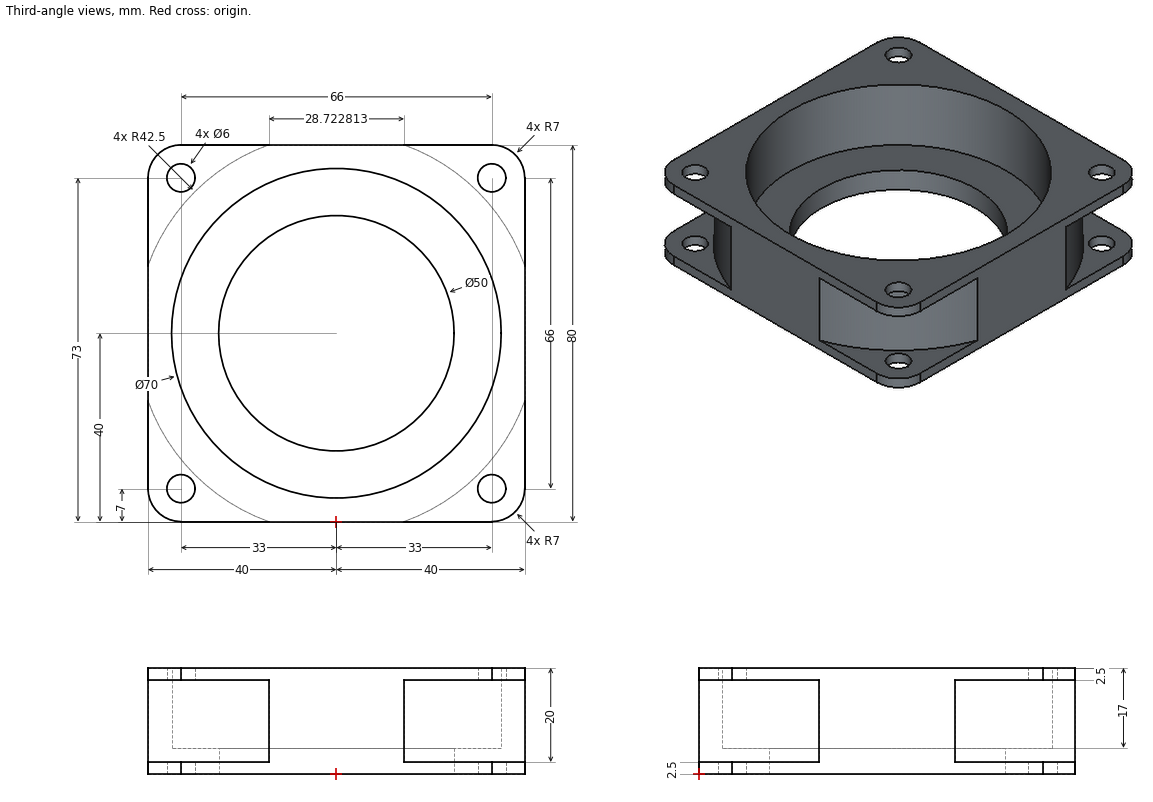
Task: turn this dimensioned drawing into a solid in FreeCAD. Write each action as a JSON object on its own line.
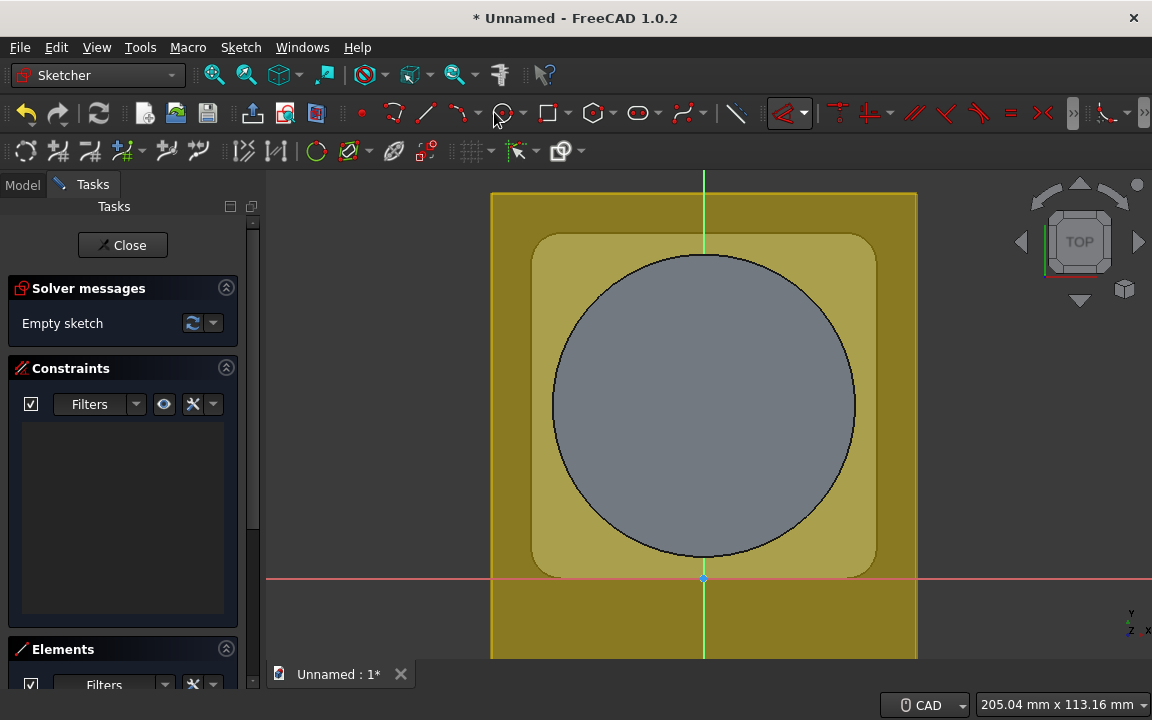
{"action": "left_click", "coordinate": [318, 114]}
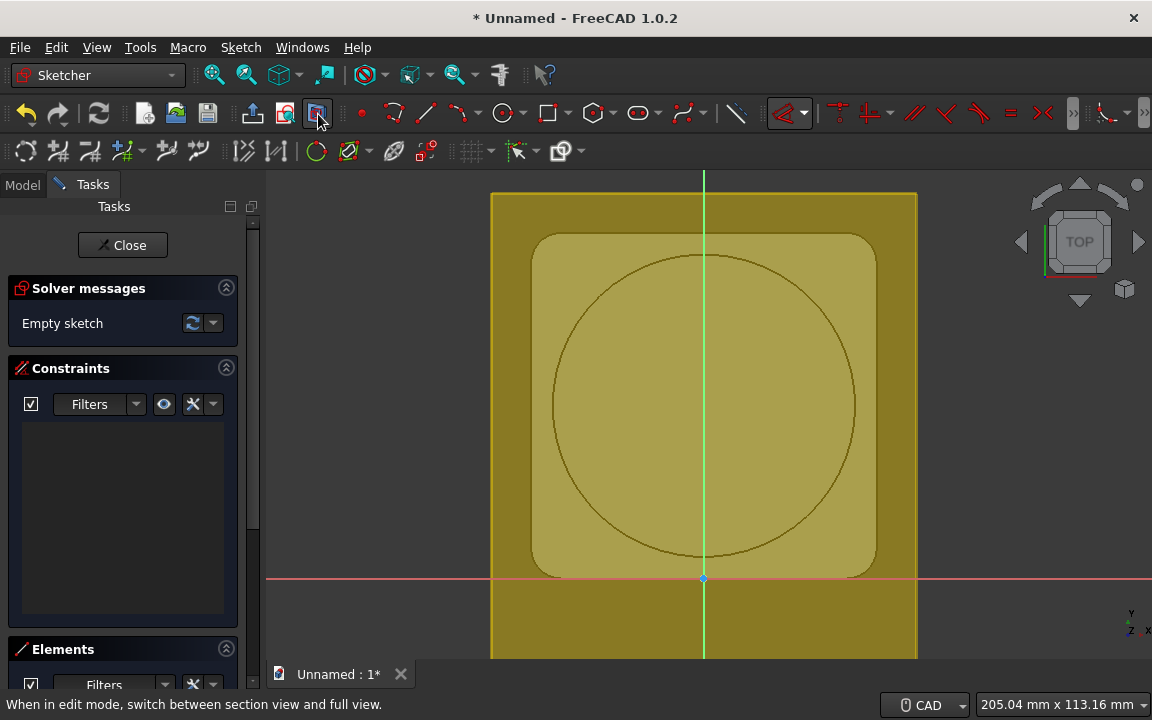
{"action": "key", "text": "g l"}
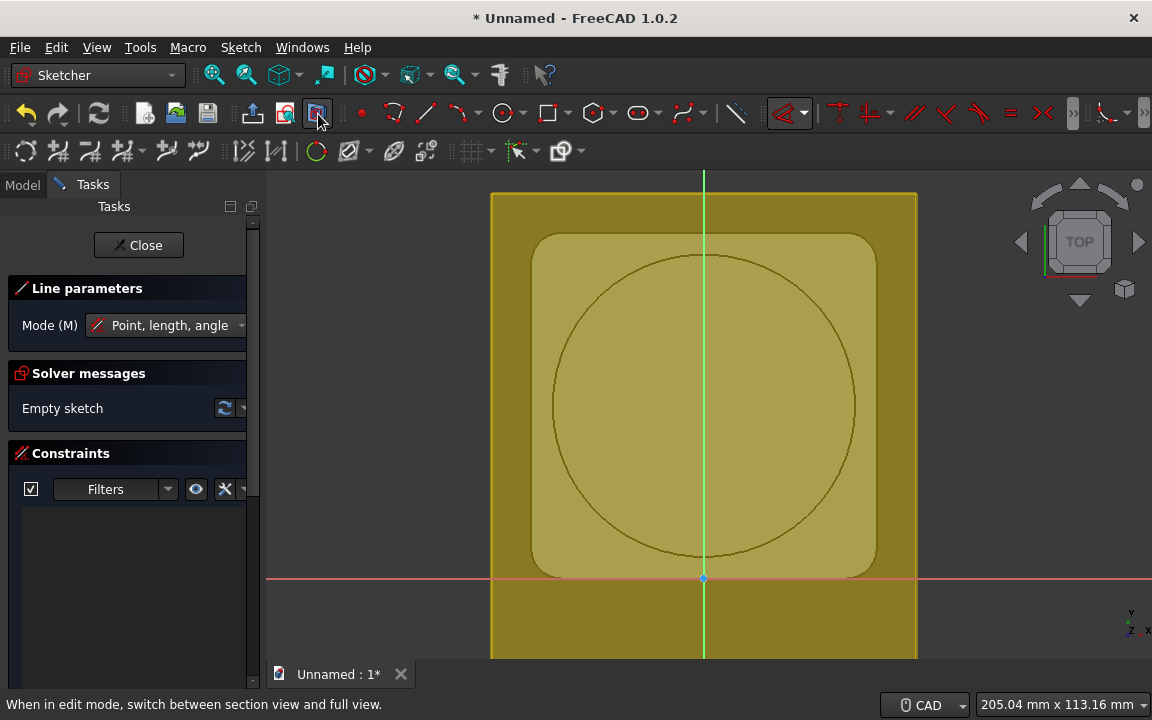
{"action": "left_click", "coordinate": [877, 548]}
{"action": "left_click", "coordinate": [877, 263]}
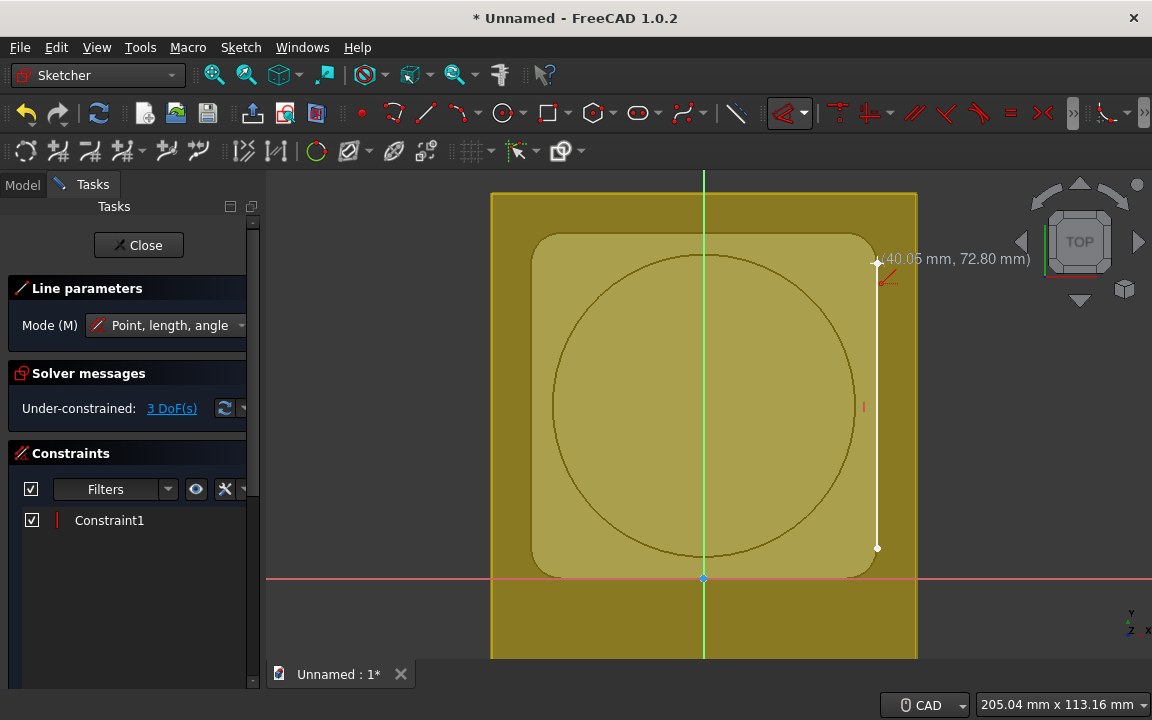
{"action": "left_click", "coordinate": [847, 233]}
{"action": "left_click", "coordinate": [561, 233]}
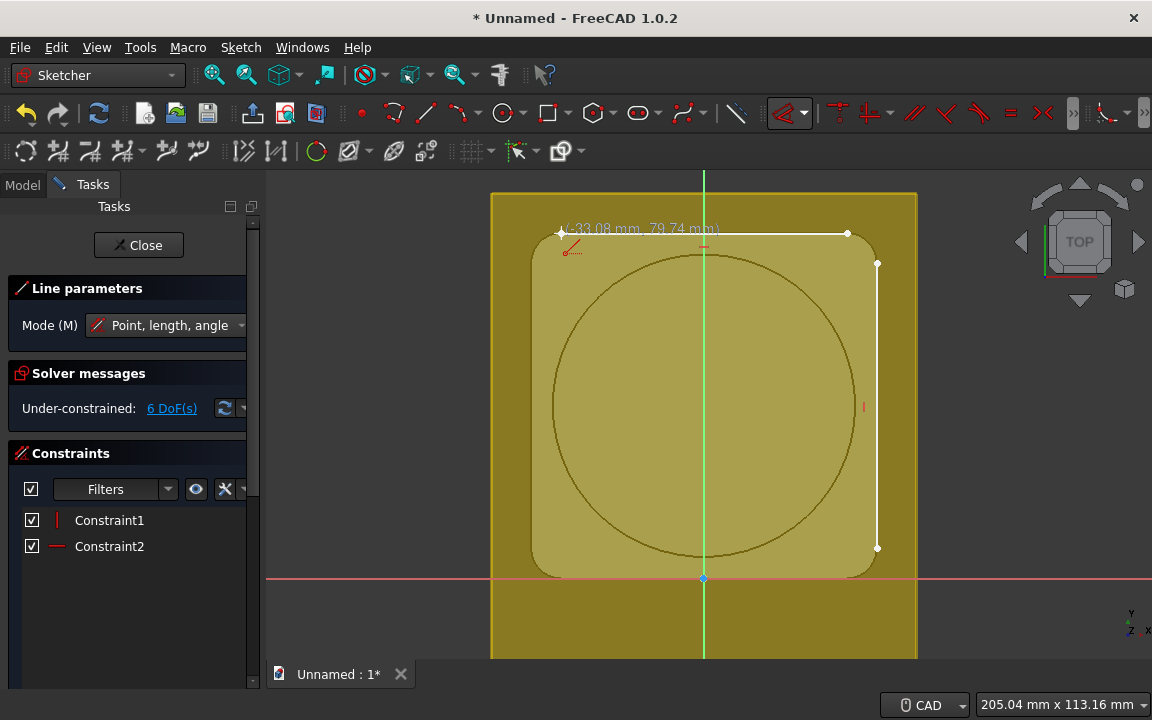
{"action": "left_click", "coordinate": [531, 263]}
{"action": "left_click", "coordinate": [531, 548]}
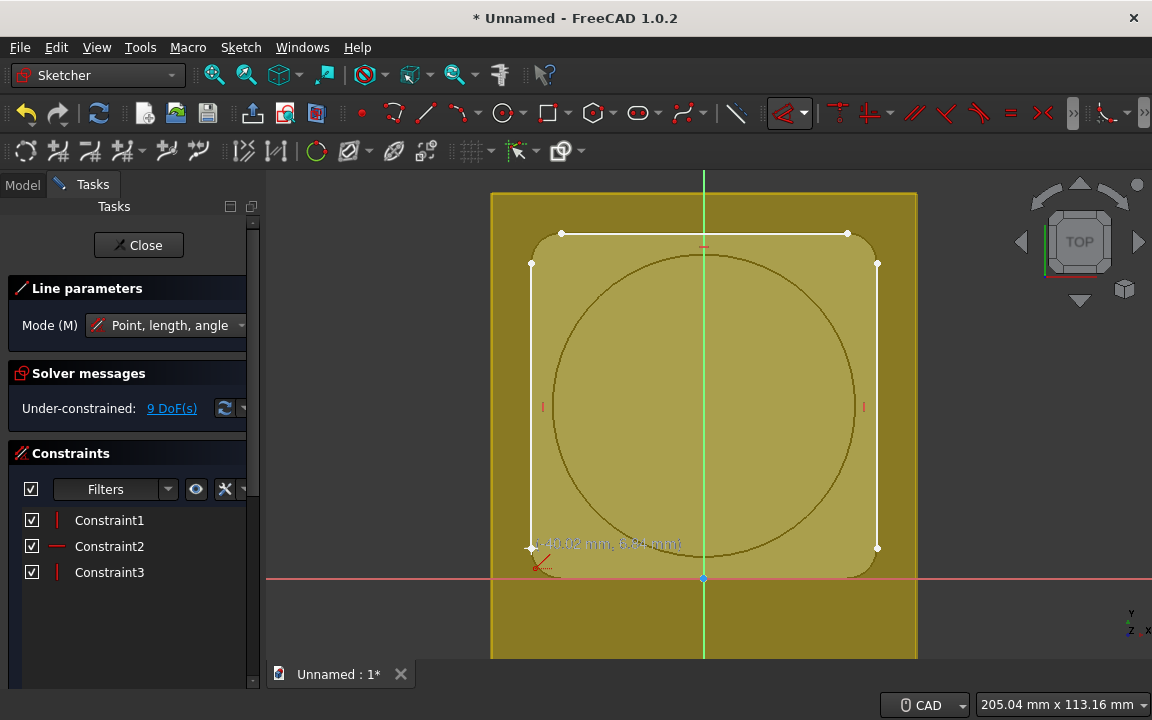
{"action": "left_click", "coordinate": [561, 579]}
{"action": "left_click", "coordinate": [847, 570]}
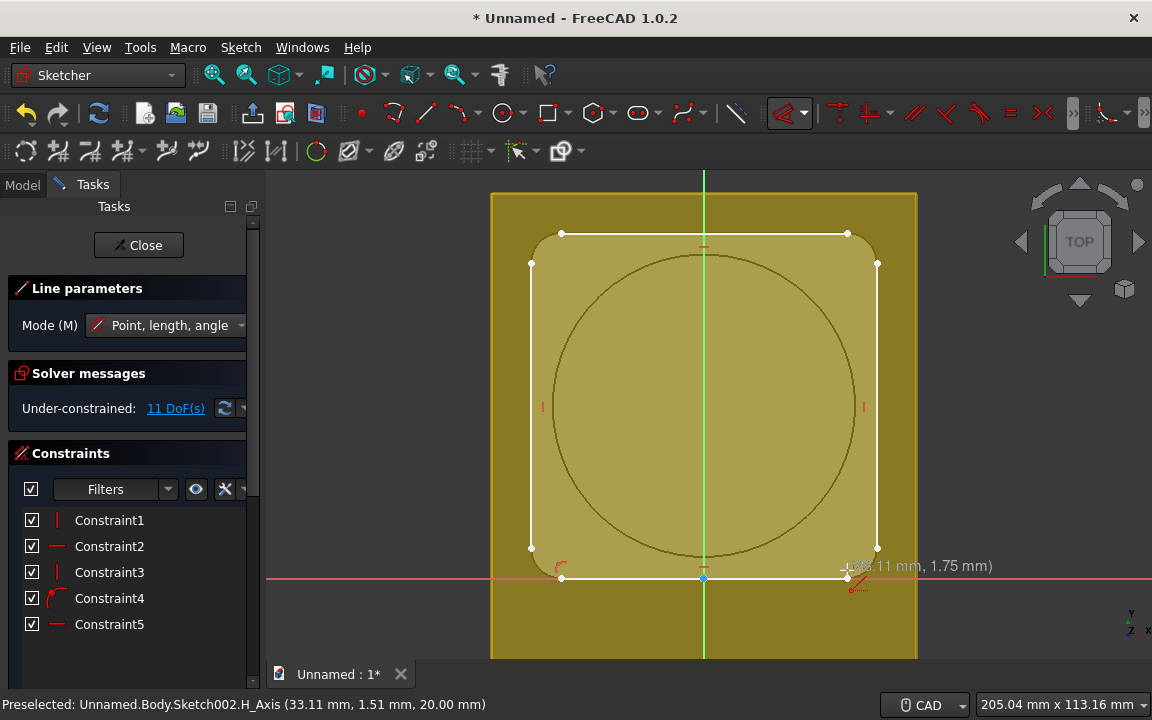
{"action": "key", "text": "g 3 a"}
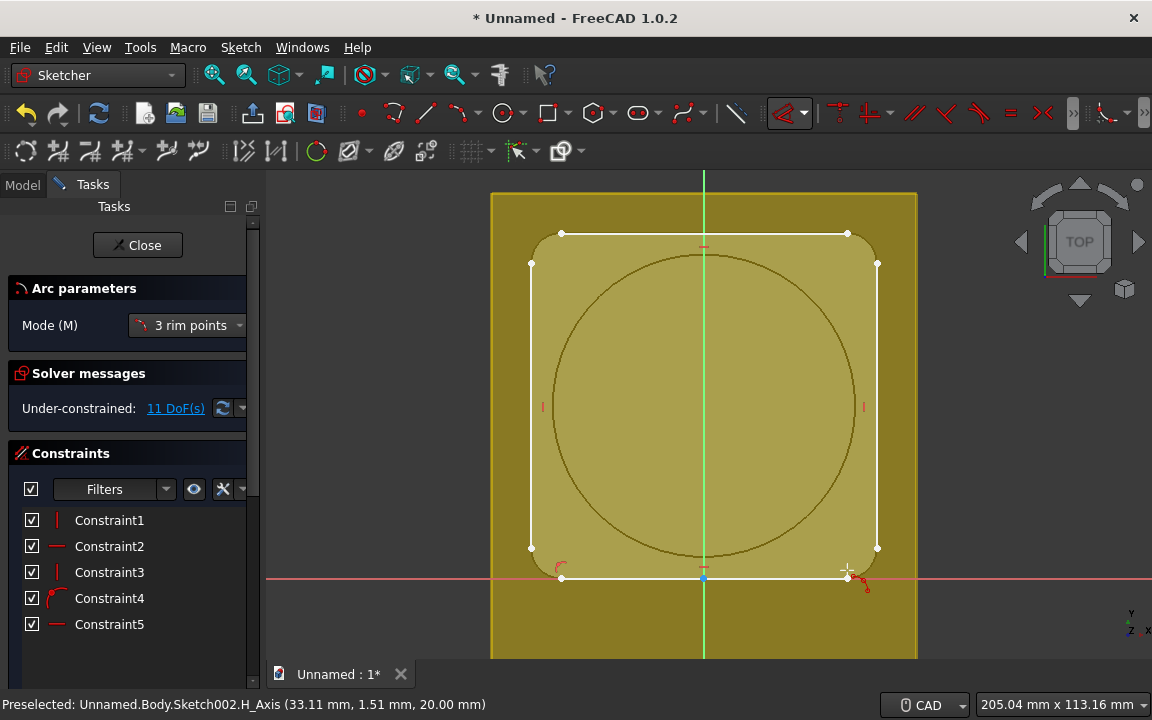
{"action": "left_click", "coordinate": [877, 264]}
{"action": "left_click", "coordinate": [847, 234]}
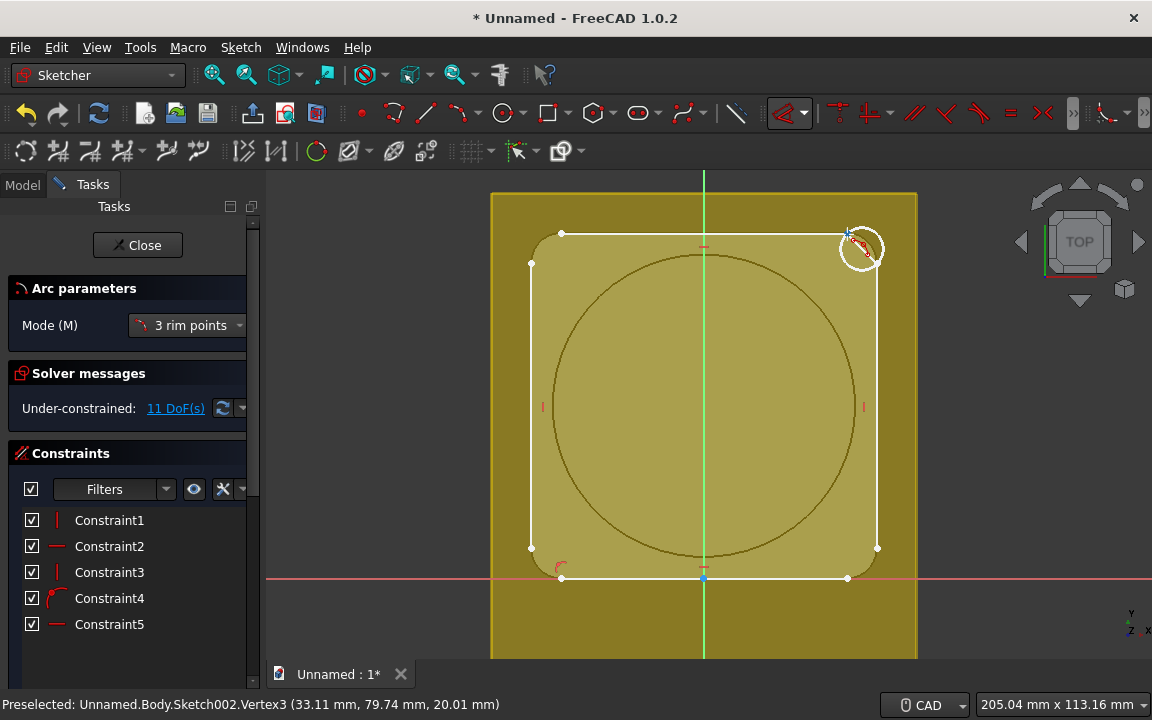
{"action": "scroll", "coordinate": [868, 242], "scroll_direction": "up", "scroll_amount": 3}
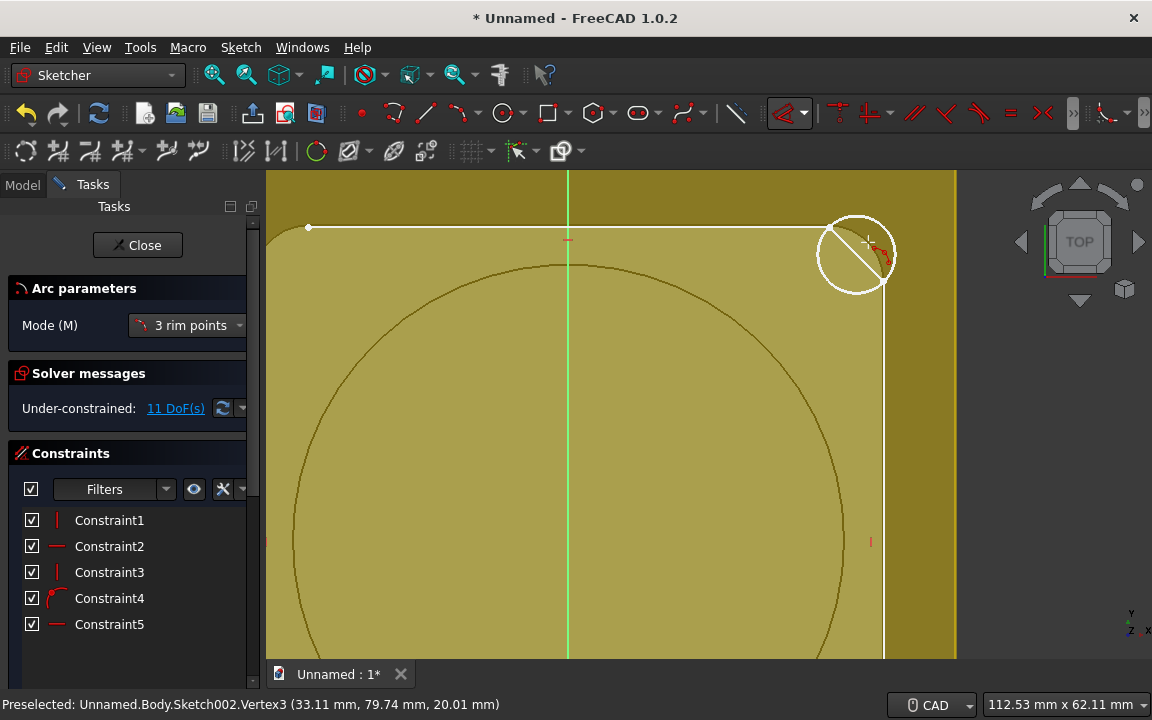
{"action": "left_click", "coordinate": [867, 241]}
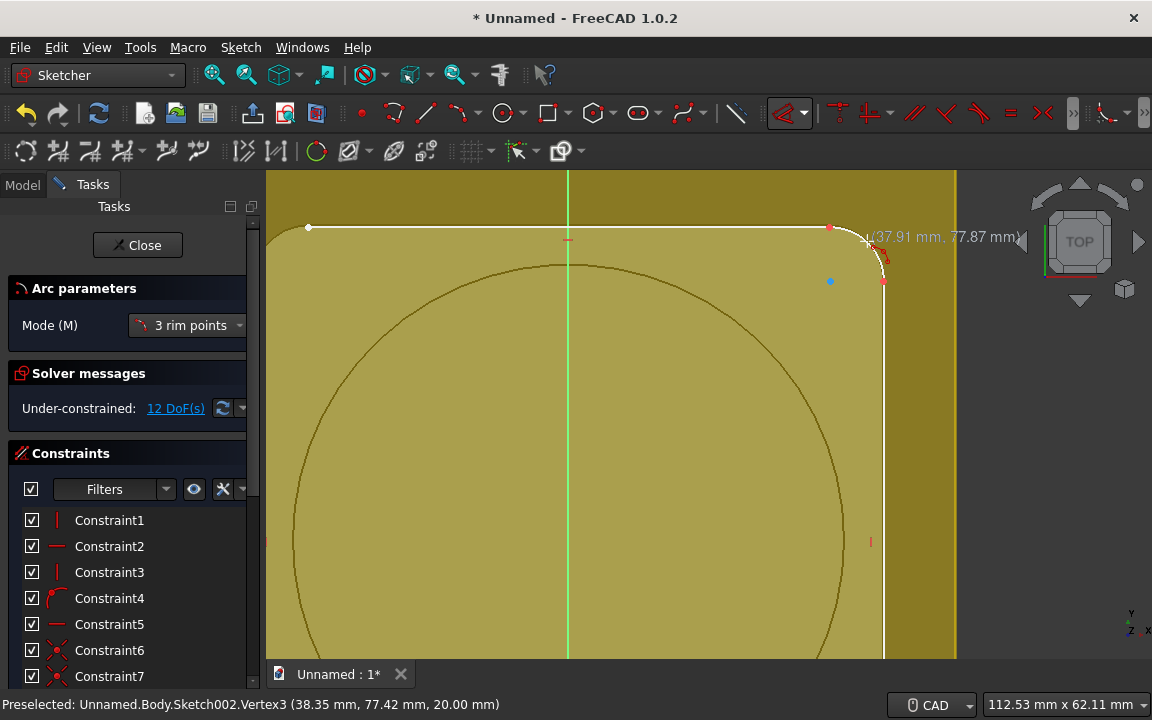
{"action": "left_click", "coordinate": [308, 227]}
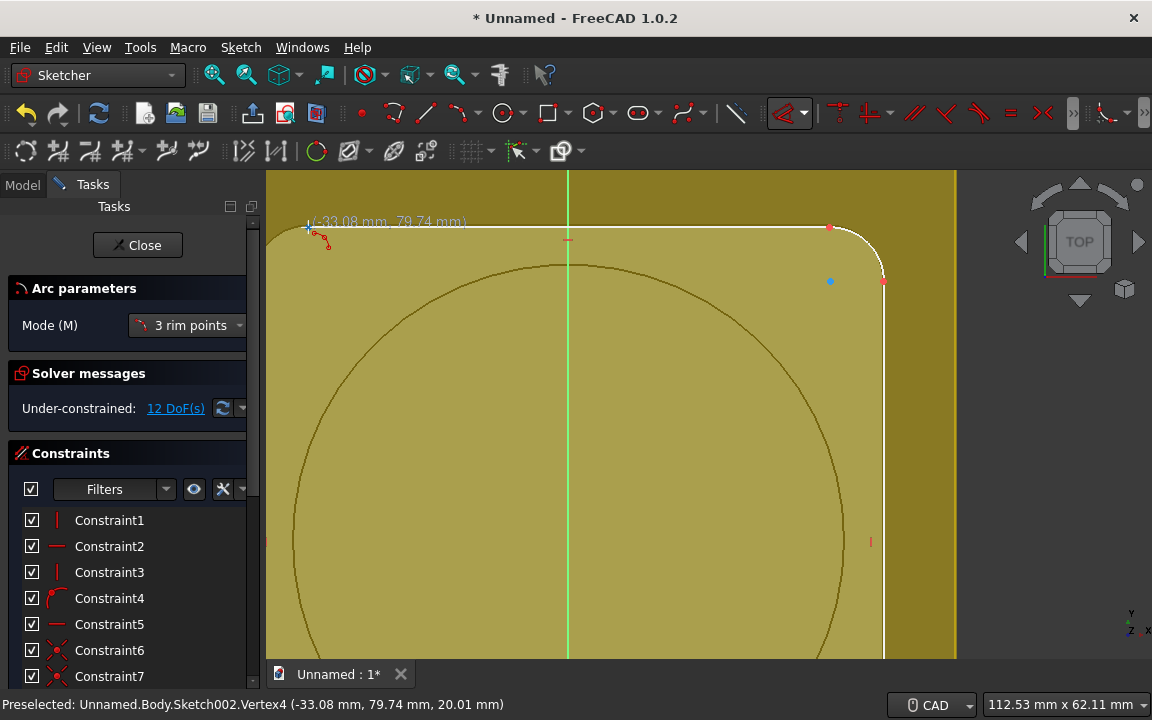
{"action": "scroll", "coordinate": [699, 312], "scroll_direction": "down", "scroll_amount": 4}